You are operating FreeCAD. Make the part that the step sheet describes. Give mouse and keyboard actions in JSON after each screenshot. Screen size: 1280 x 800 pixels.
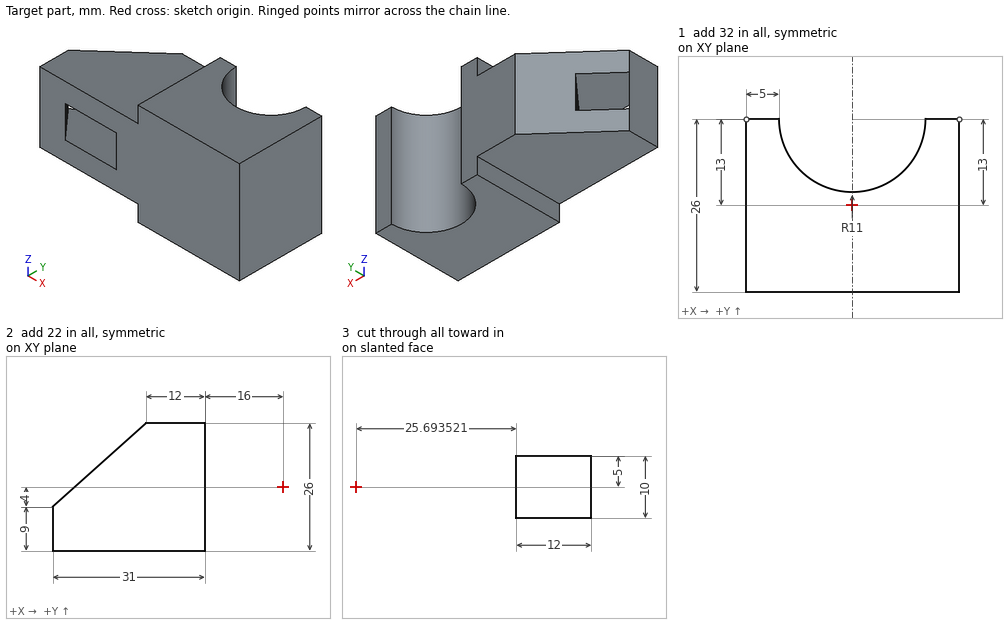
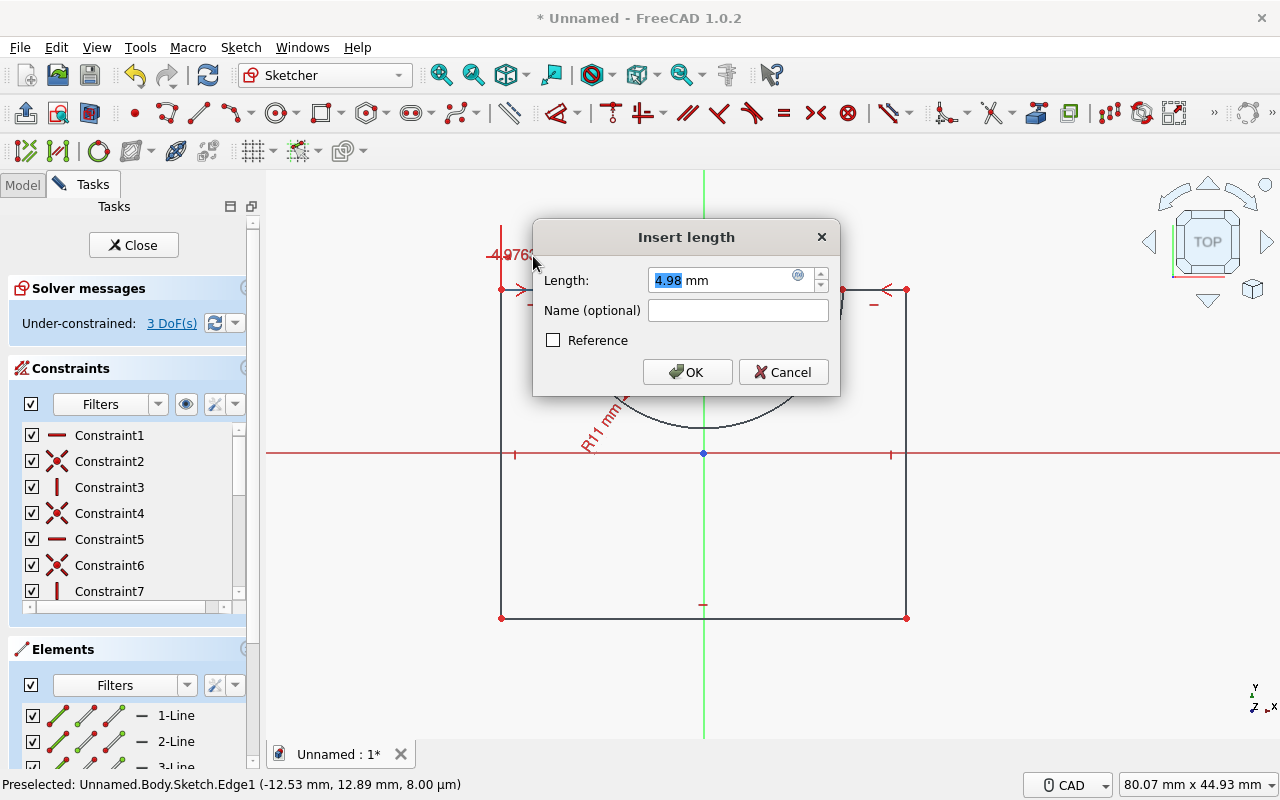
{"action": "type", "text": "5"}
{"action": "key", "text": "Return"}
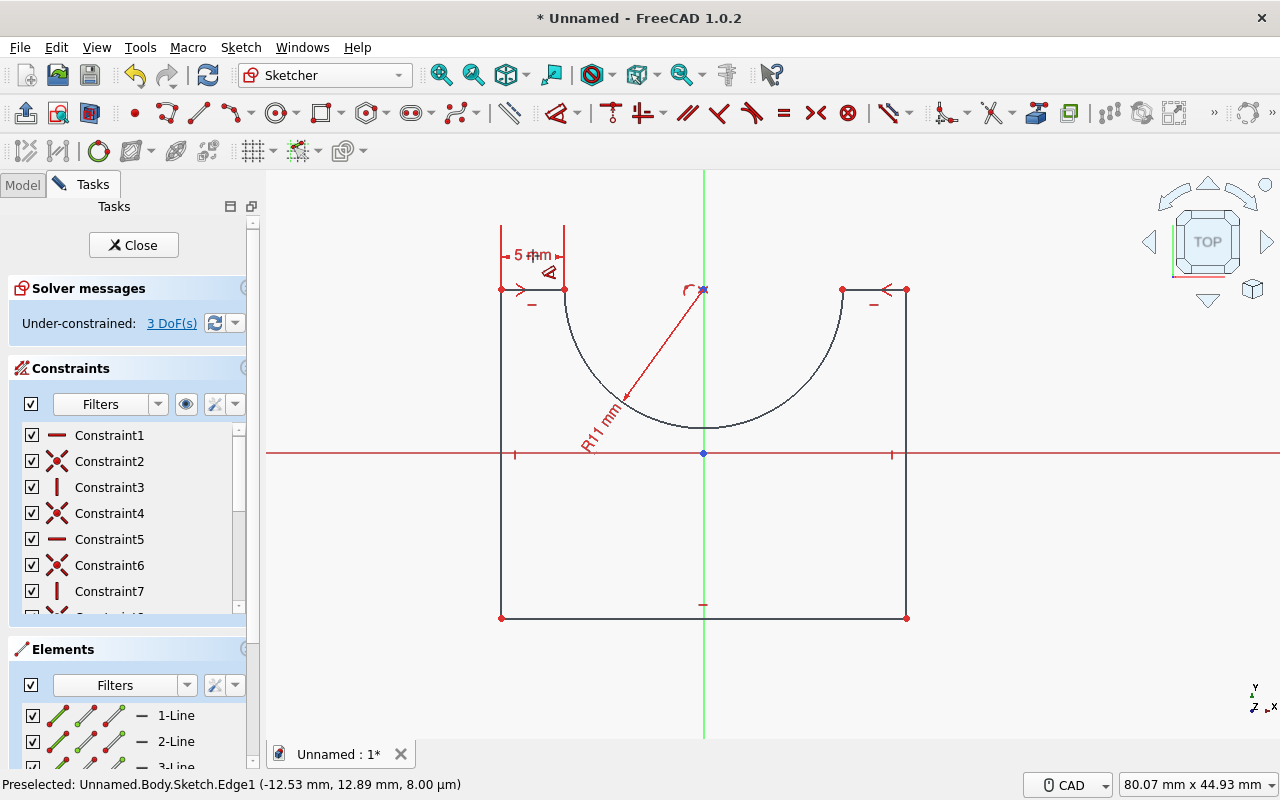
{"action": "left_click", "coordinate": [501, 389]}
{"action": "left_click", "coordinate": [467, 379]}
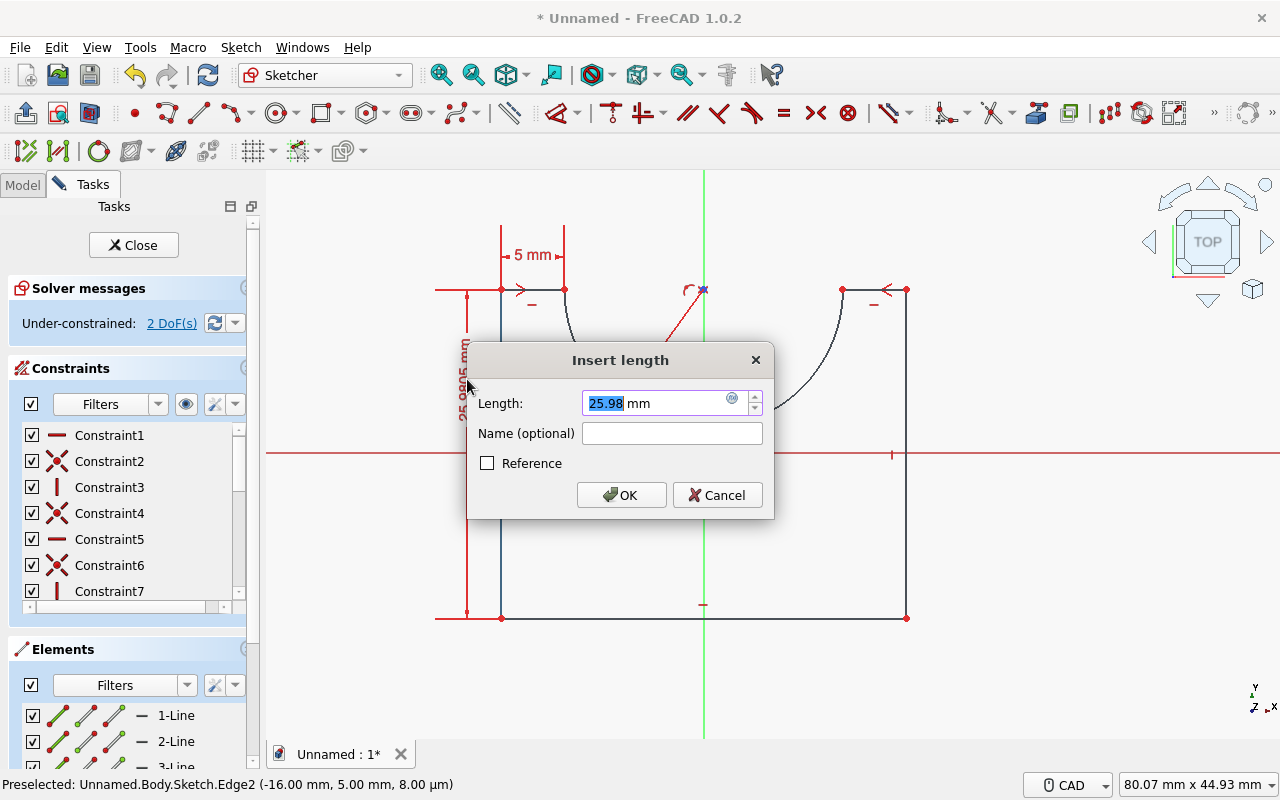
{"action": "type", "text": "26"}
{"action": "key", "text": "Return"}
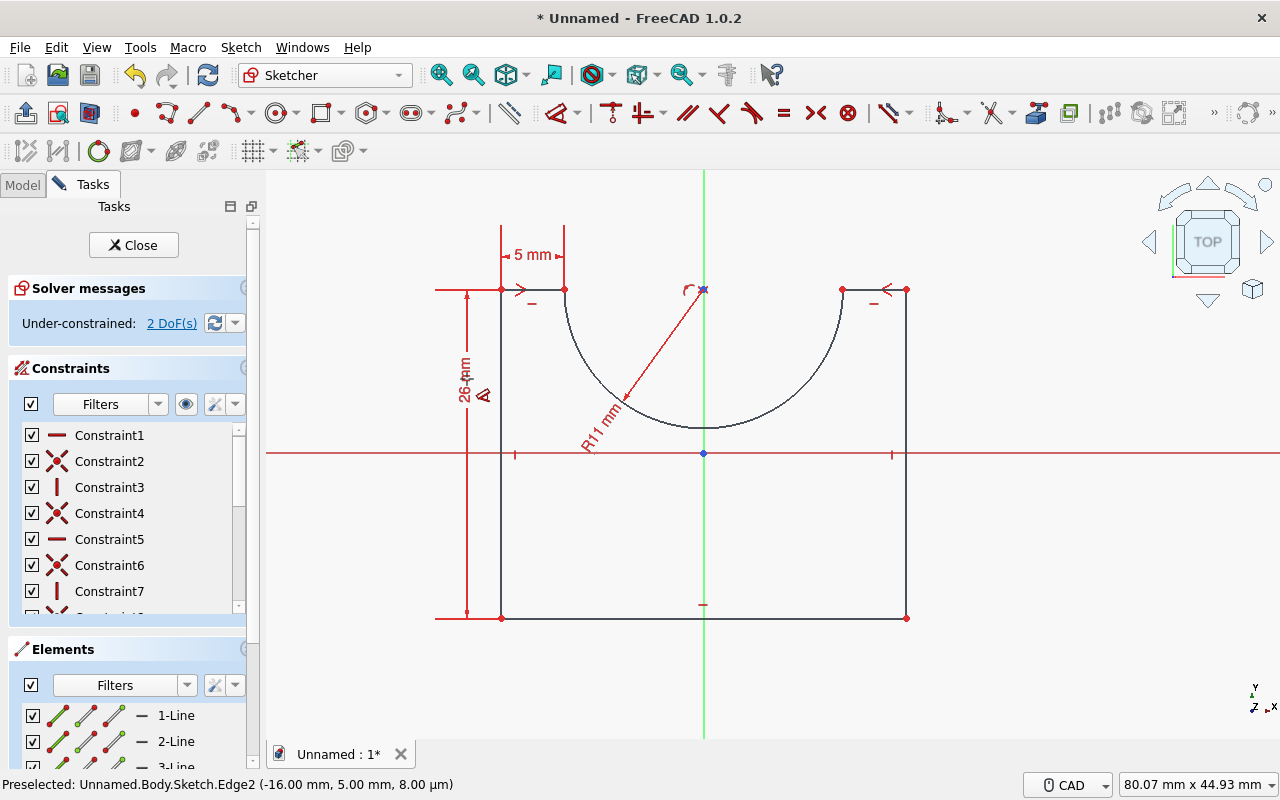
{"action": "left_click", "coordinate": [564, 290]}
{"action": "left_click", "coordinate": [530, 334]}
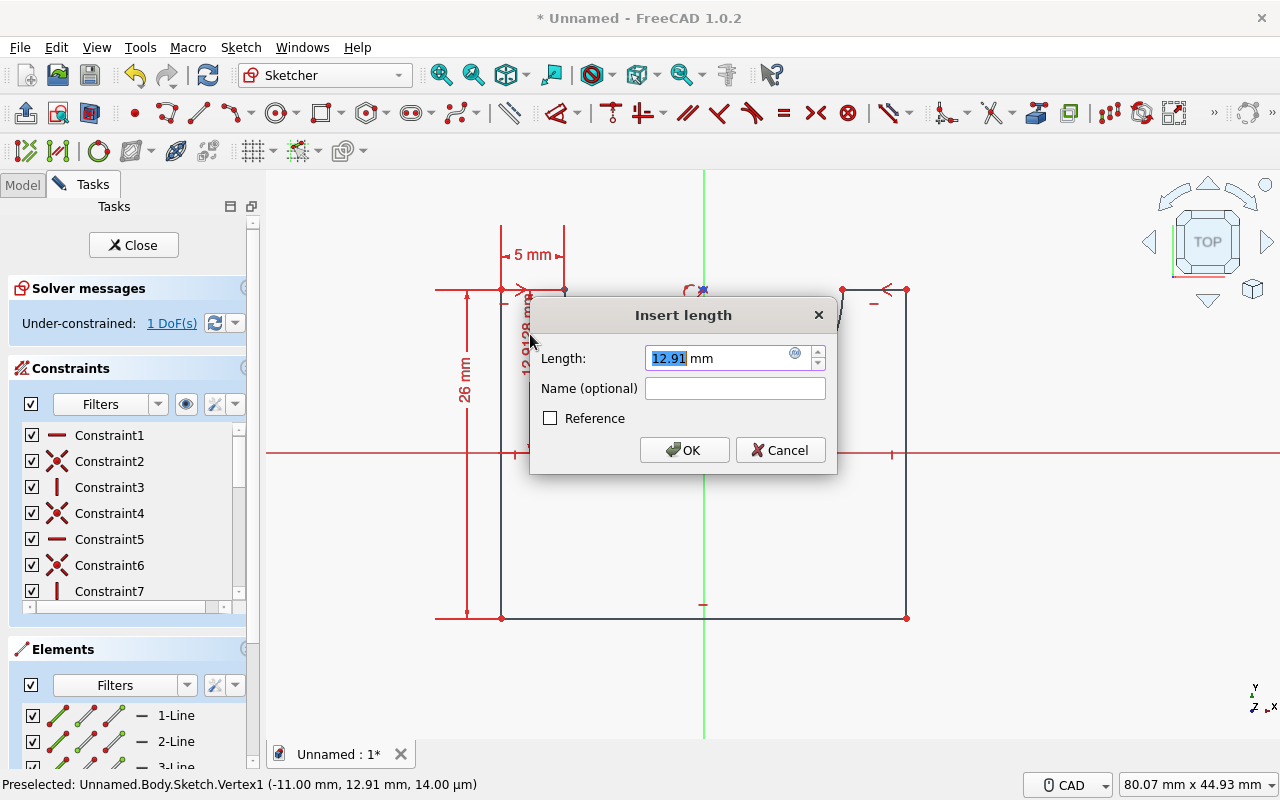
{"action": "type", "text": "13"}
{"action": "key", "text": "Return"}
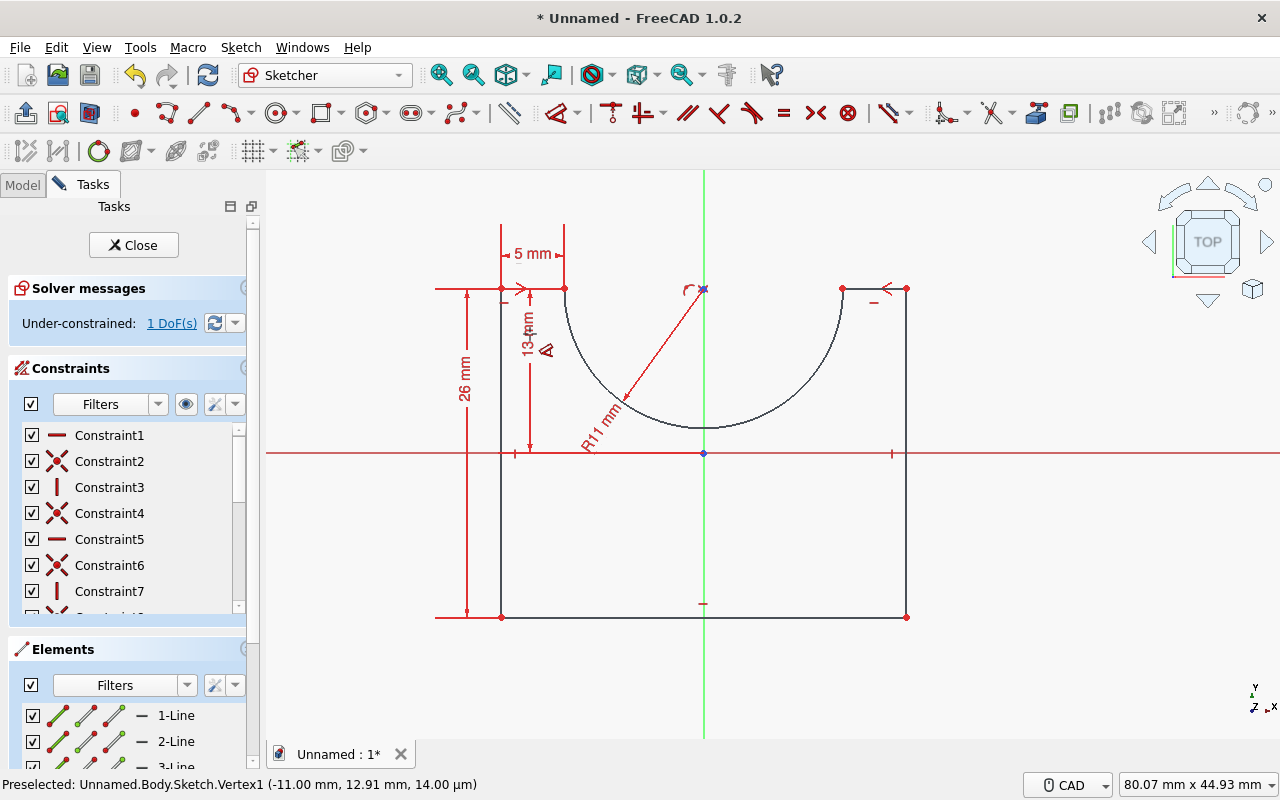
{"action": "left_click", "coordinate": [704, 289]}
{"action": "left_click", "coordinate": [738, 371]}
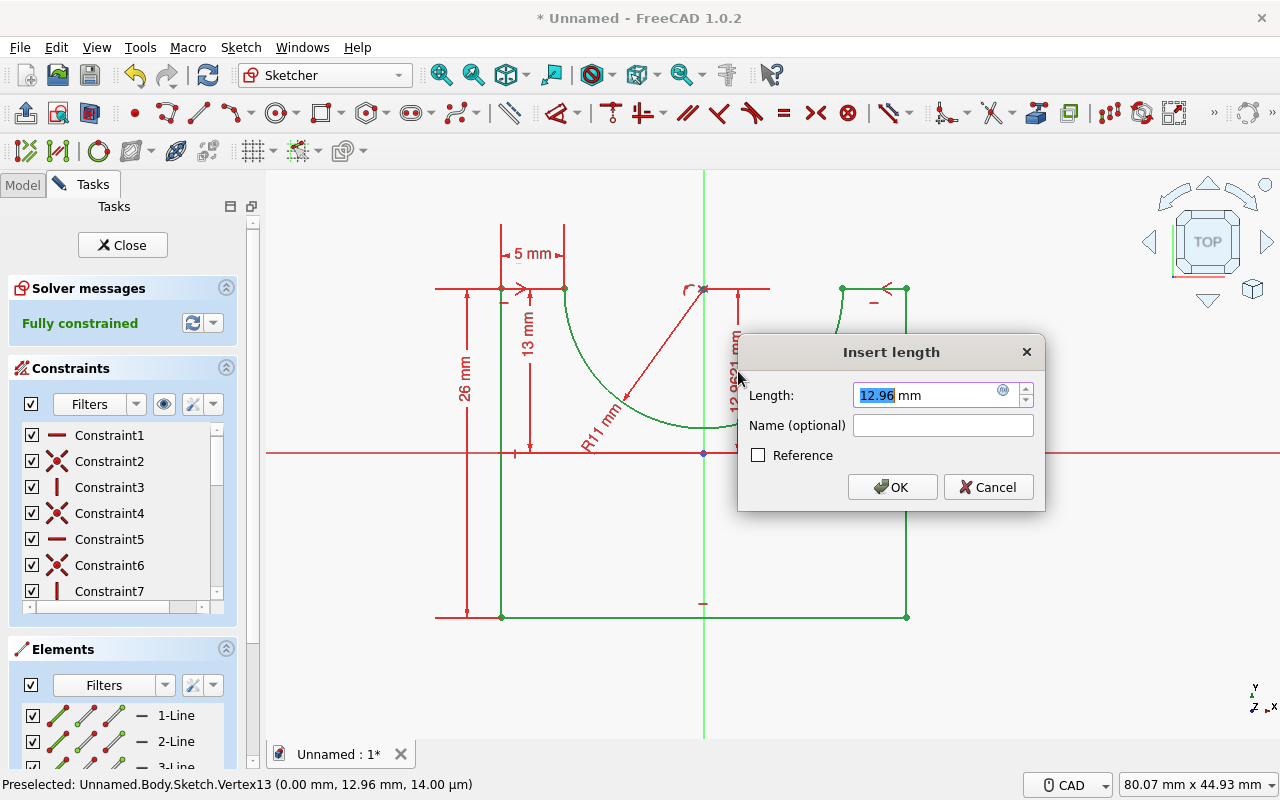
{"action": "type", "text": "13"}
{"action": "key", "text": "Return"}
{"action": "key", "text": "Escape"}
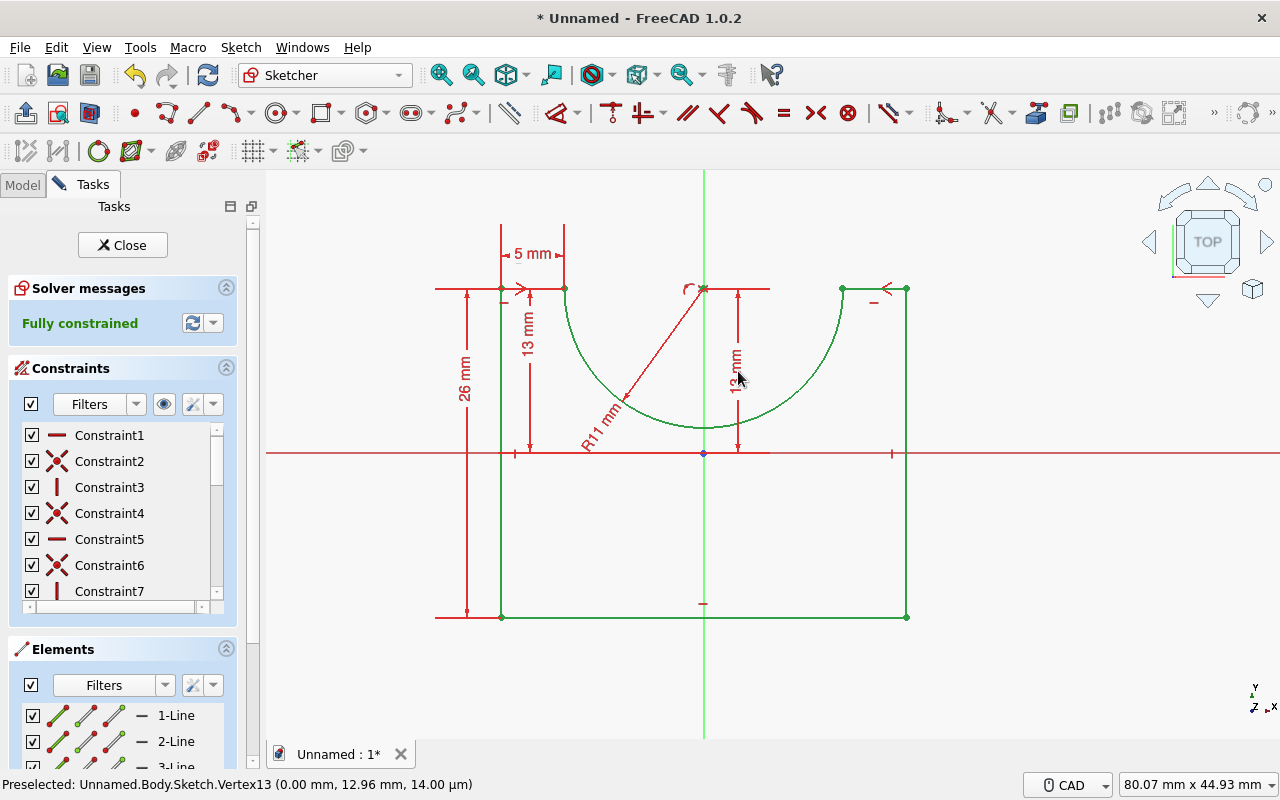
{"action": "left_click", "coordinate": [123, 245]}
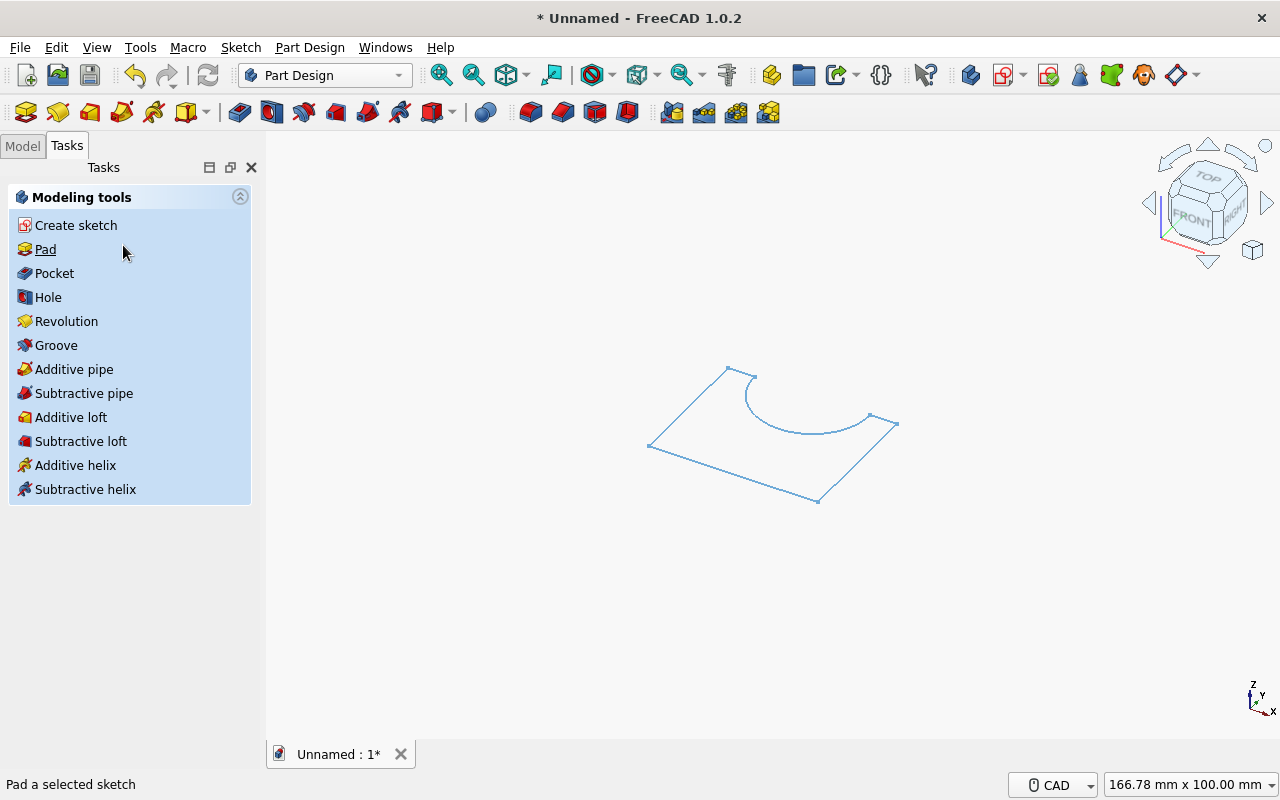
{"action": "left_click", "coordinate": [26, 112]}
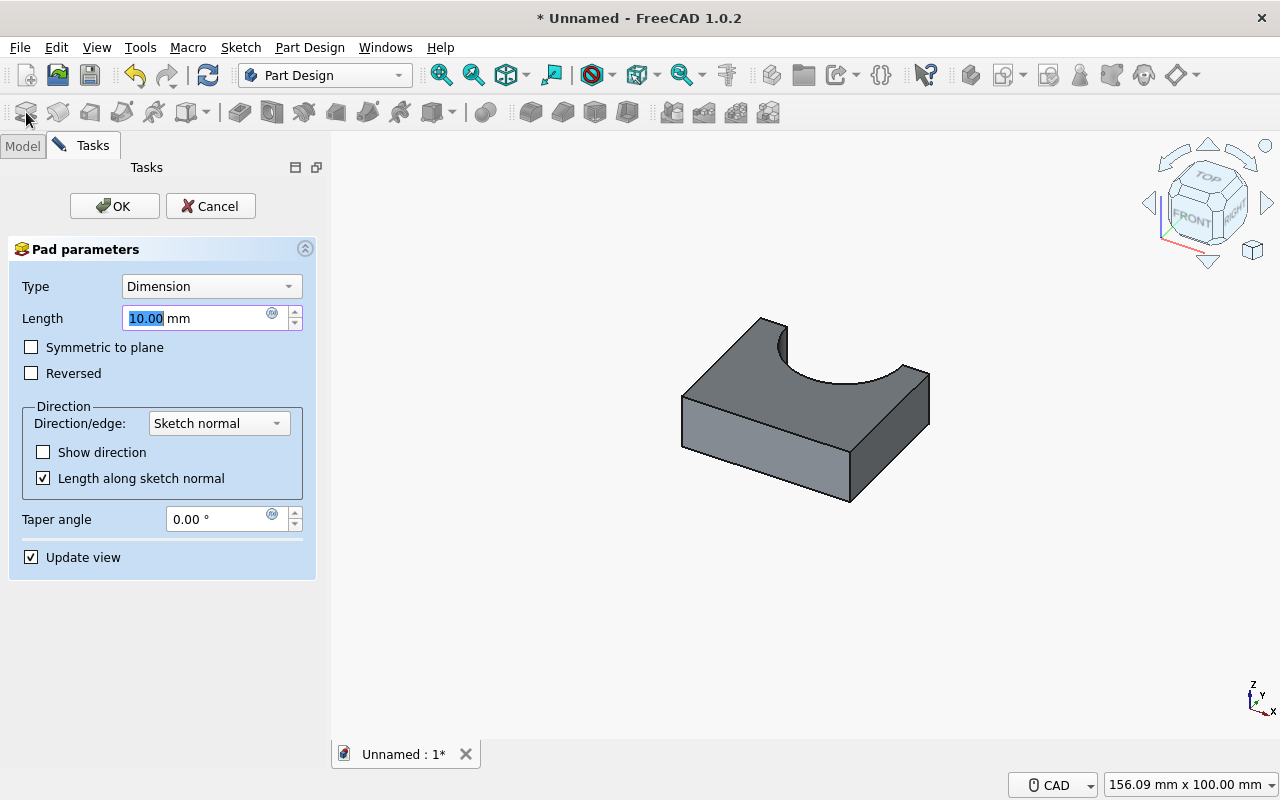
{"action": "type", "text": "32"}
{"action": "key", "text": "Tab"}